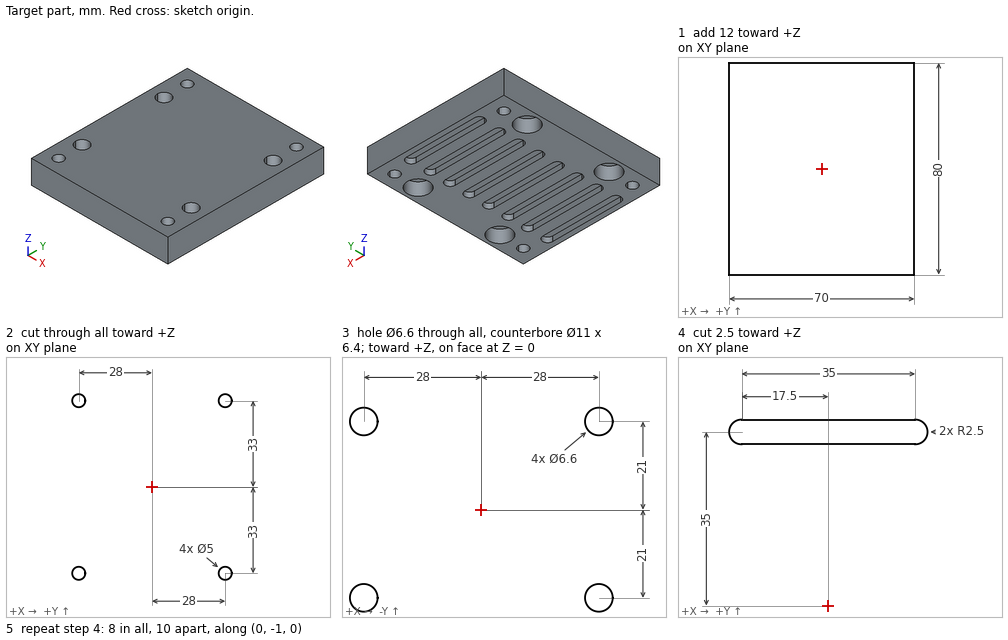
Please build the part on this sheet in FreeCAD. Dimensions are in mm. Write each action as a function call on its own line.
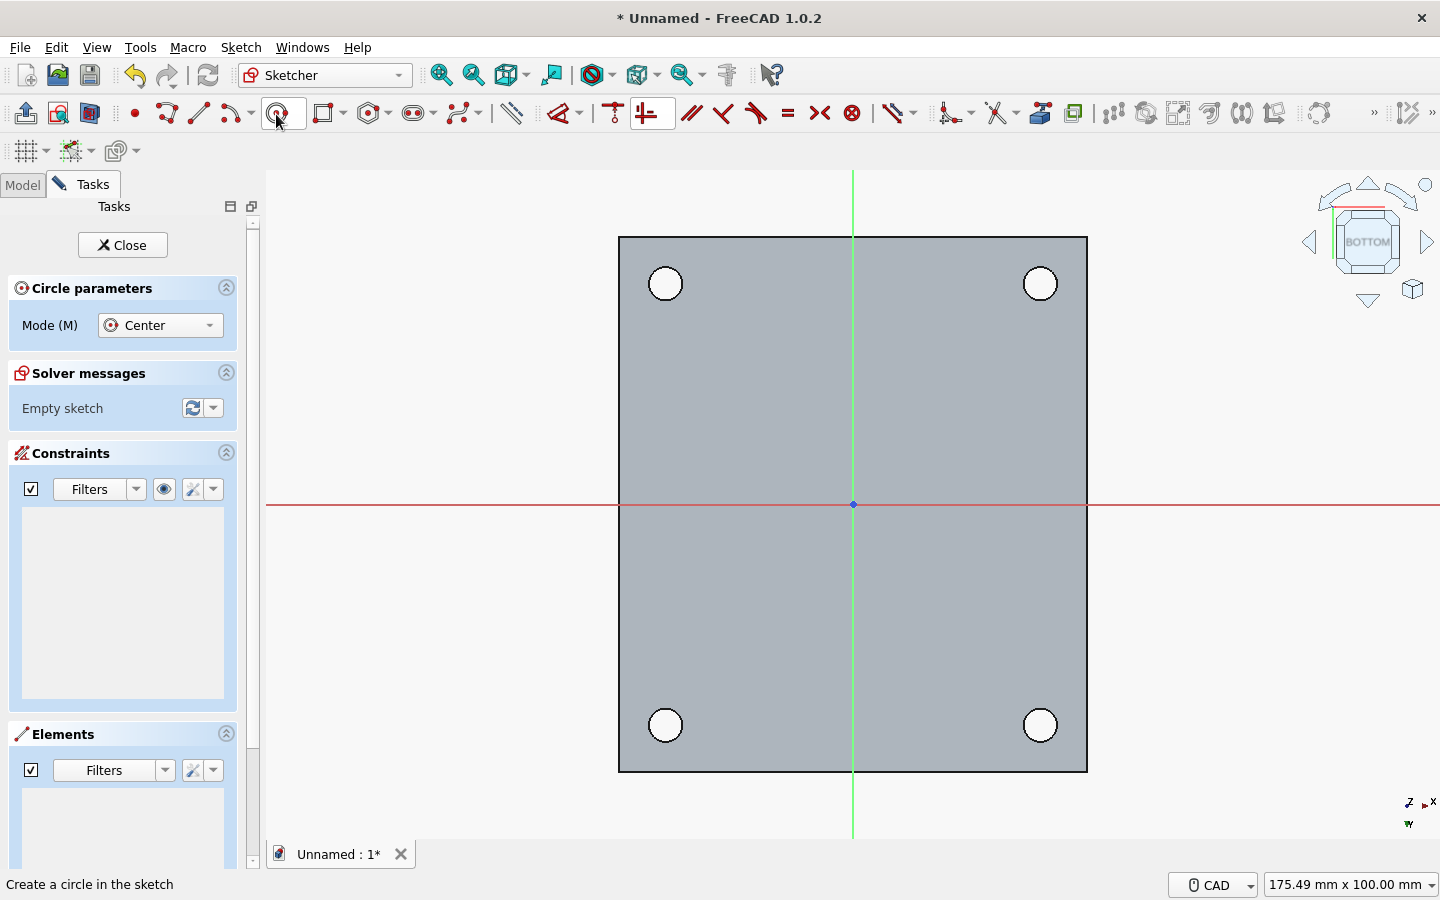
click(1040, 364)
move(1056, 348)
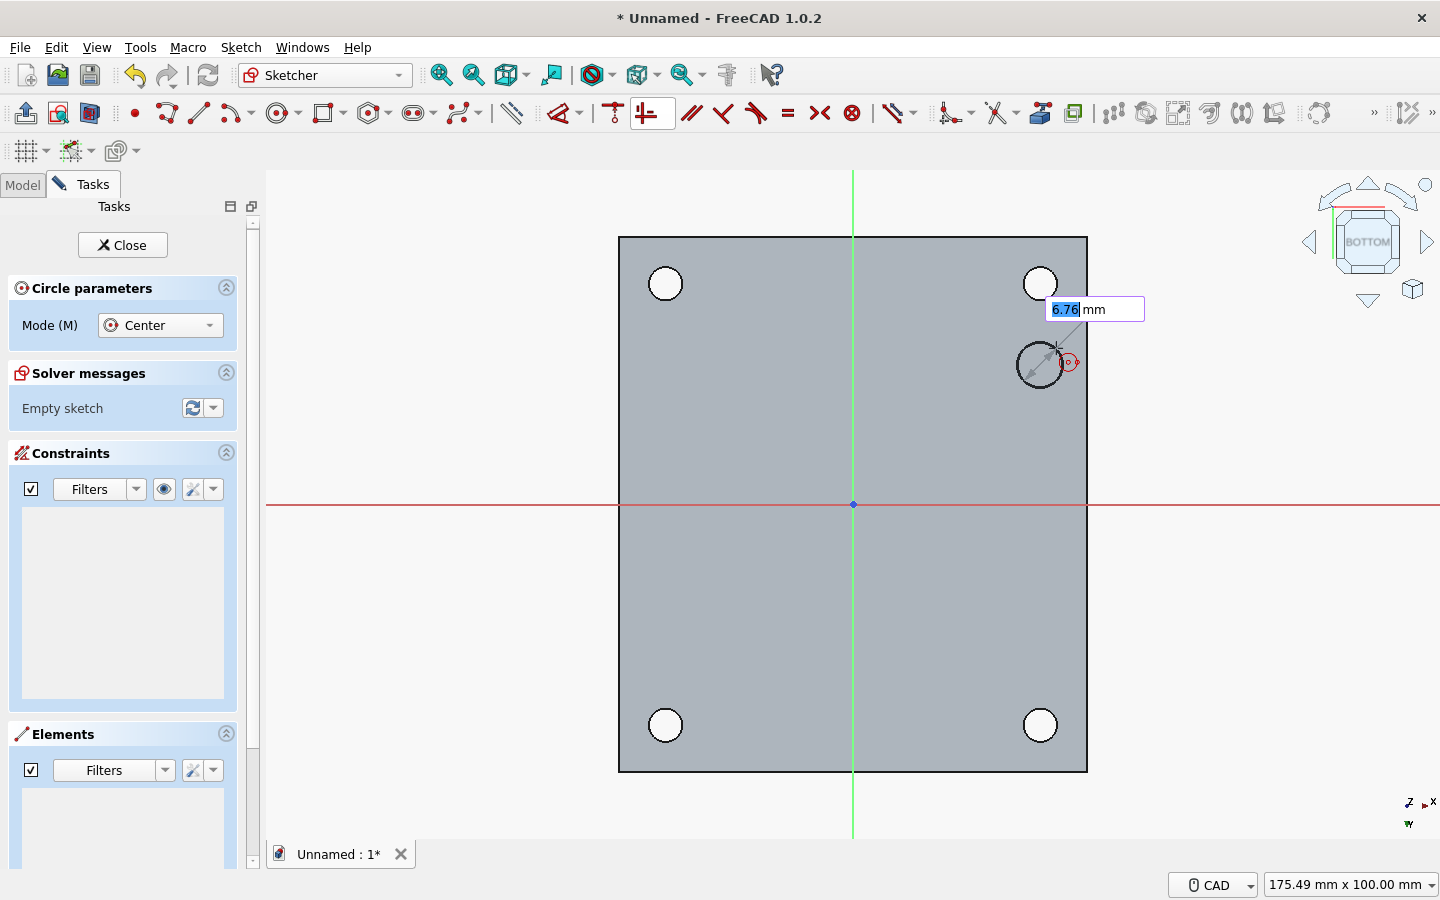
text(6.6)
key(Return)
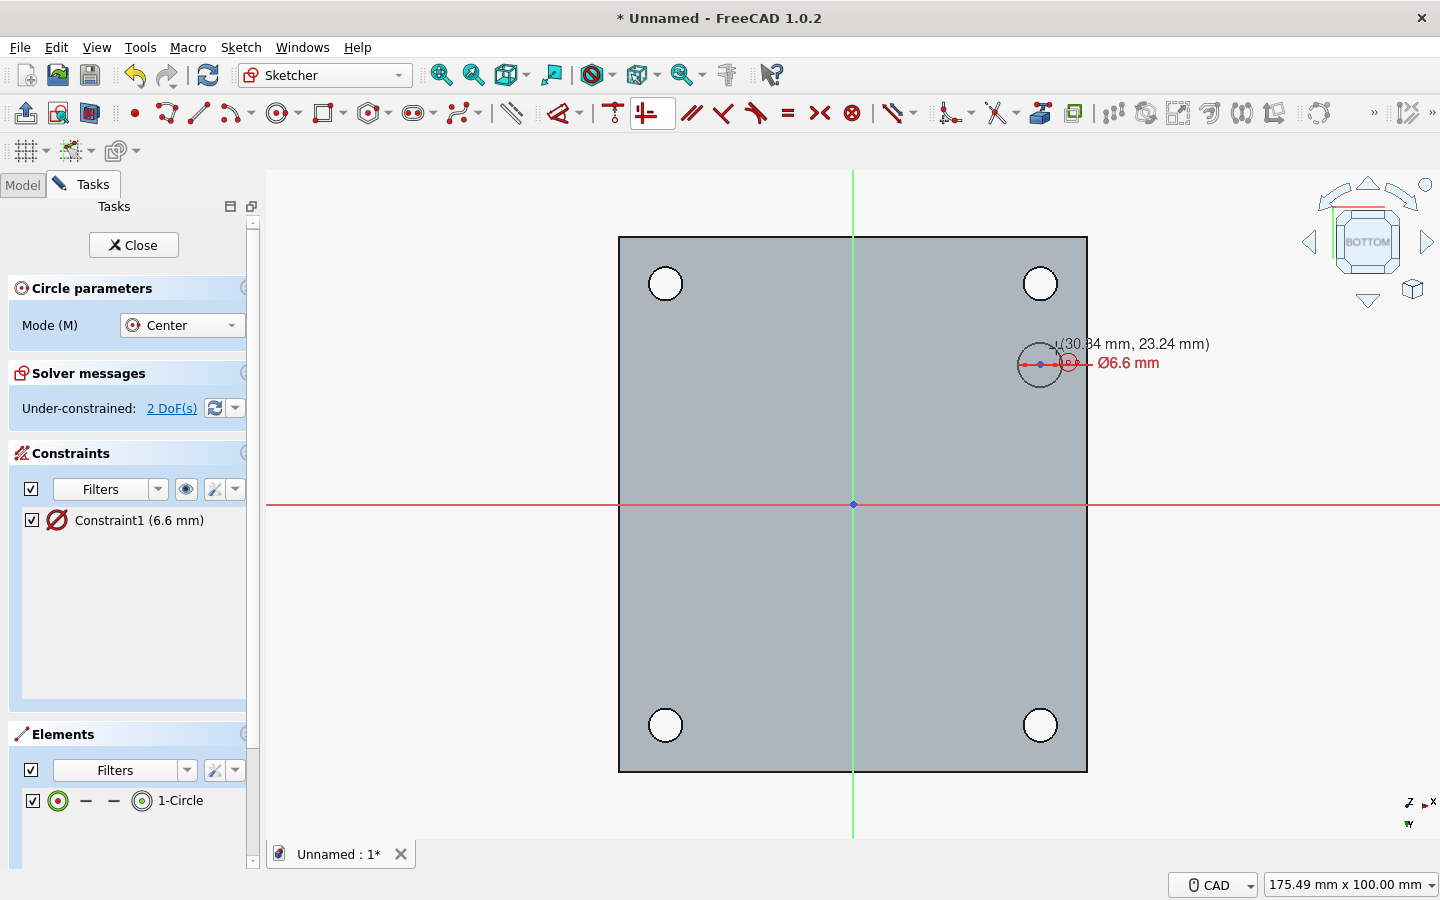
click(1040, 645)
move(1056, 629)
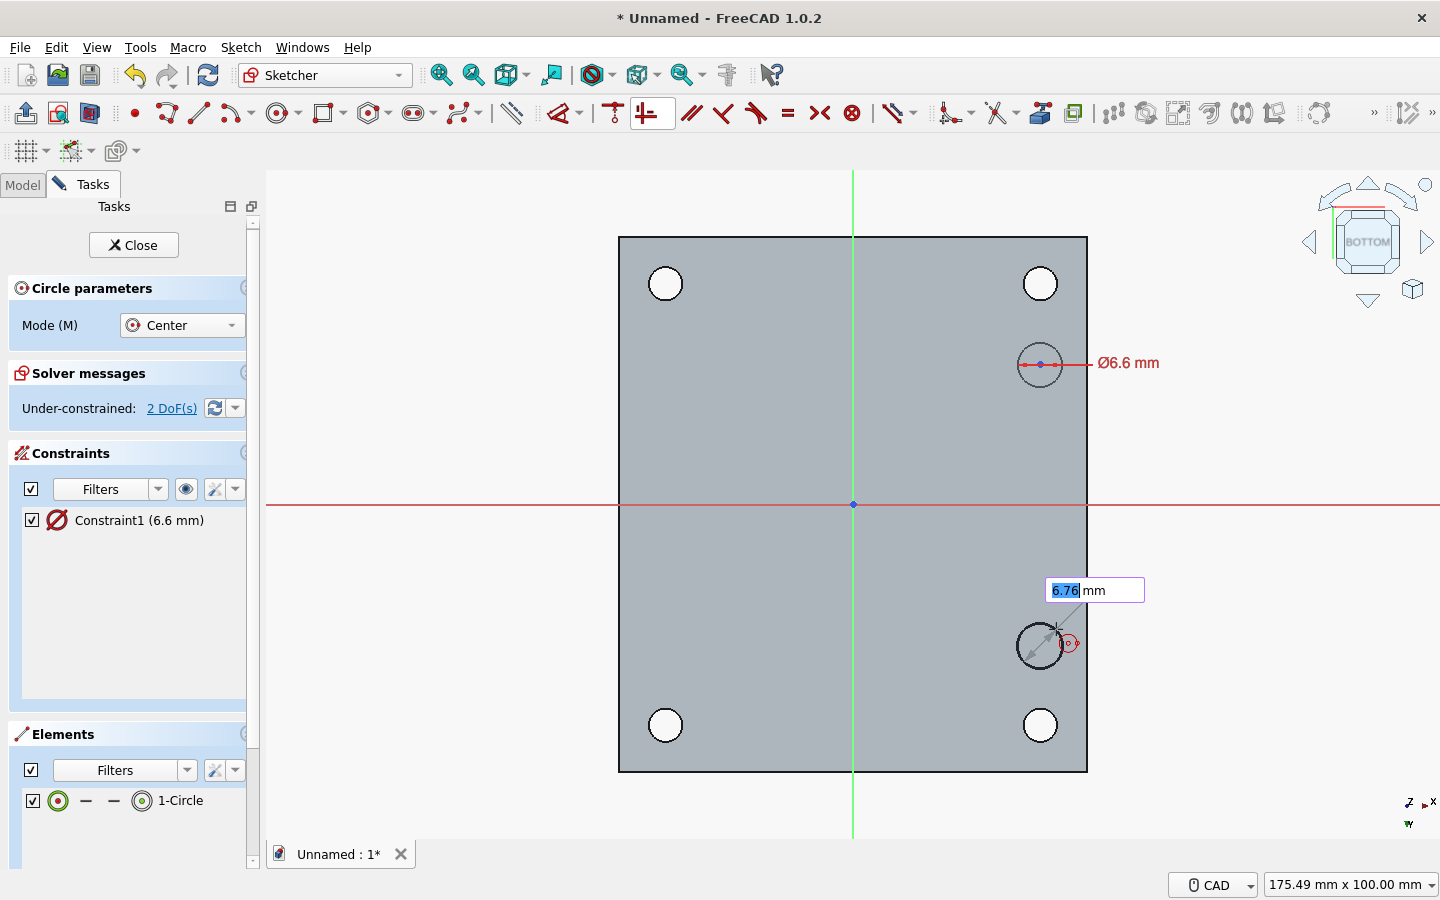
text(6.6)
key(Return)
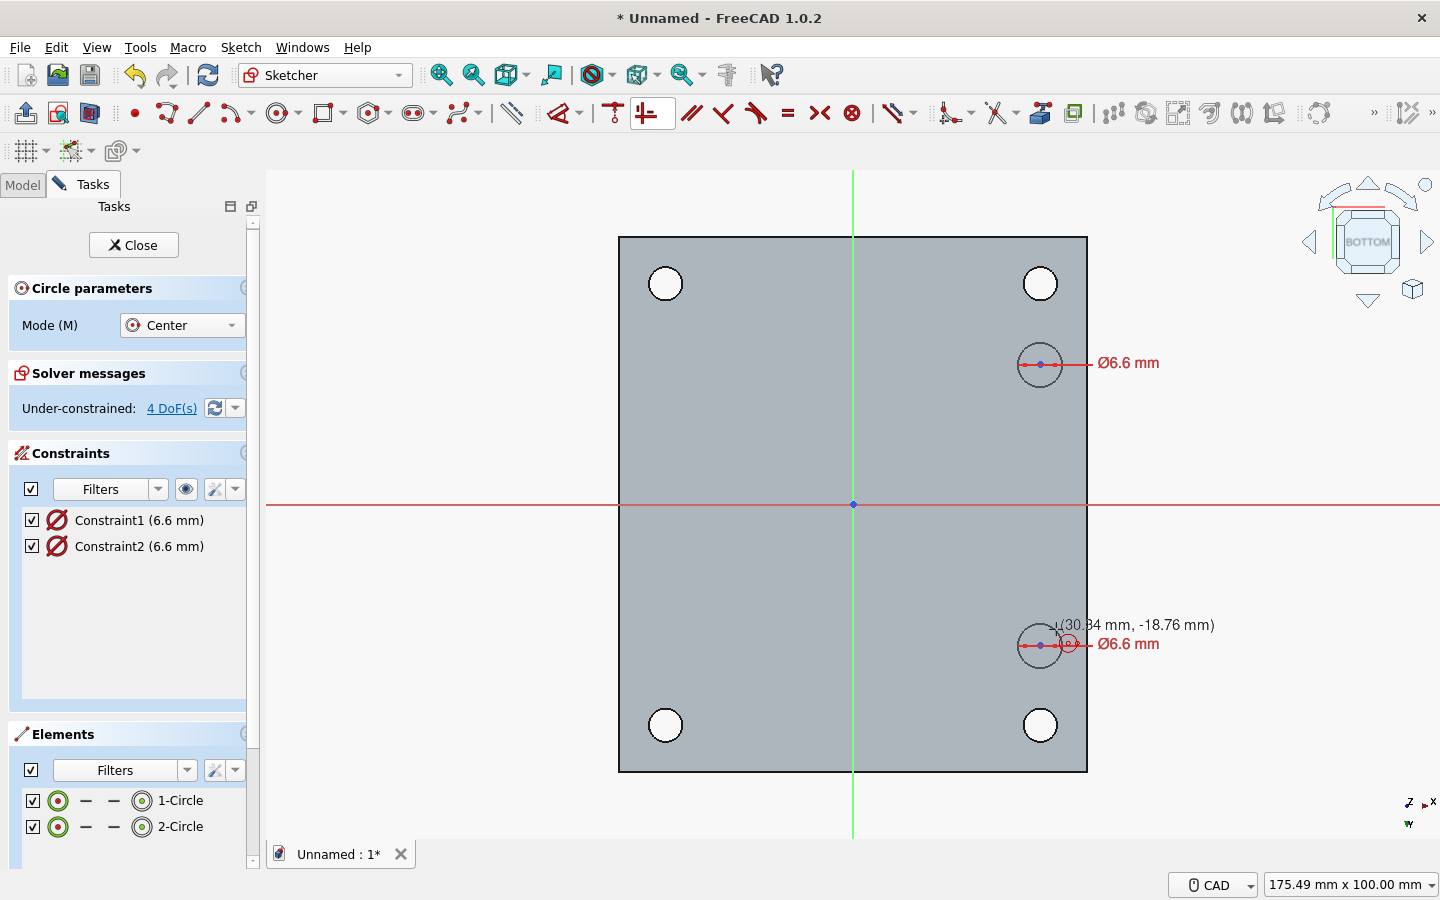
click(666, 364)
move(681, 348)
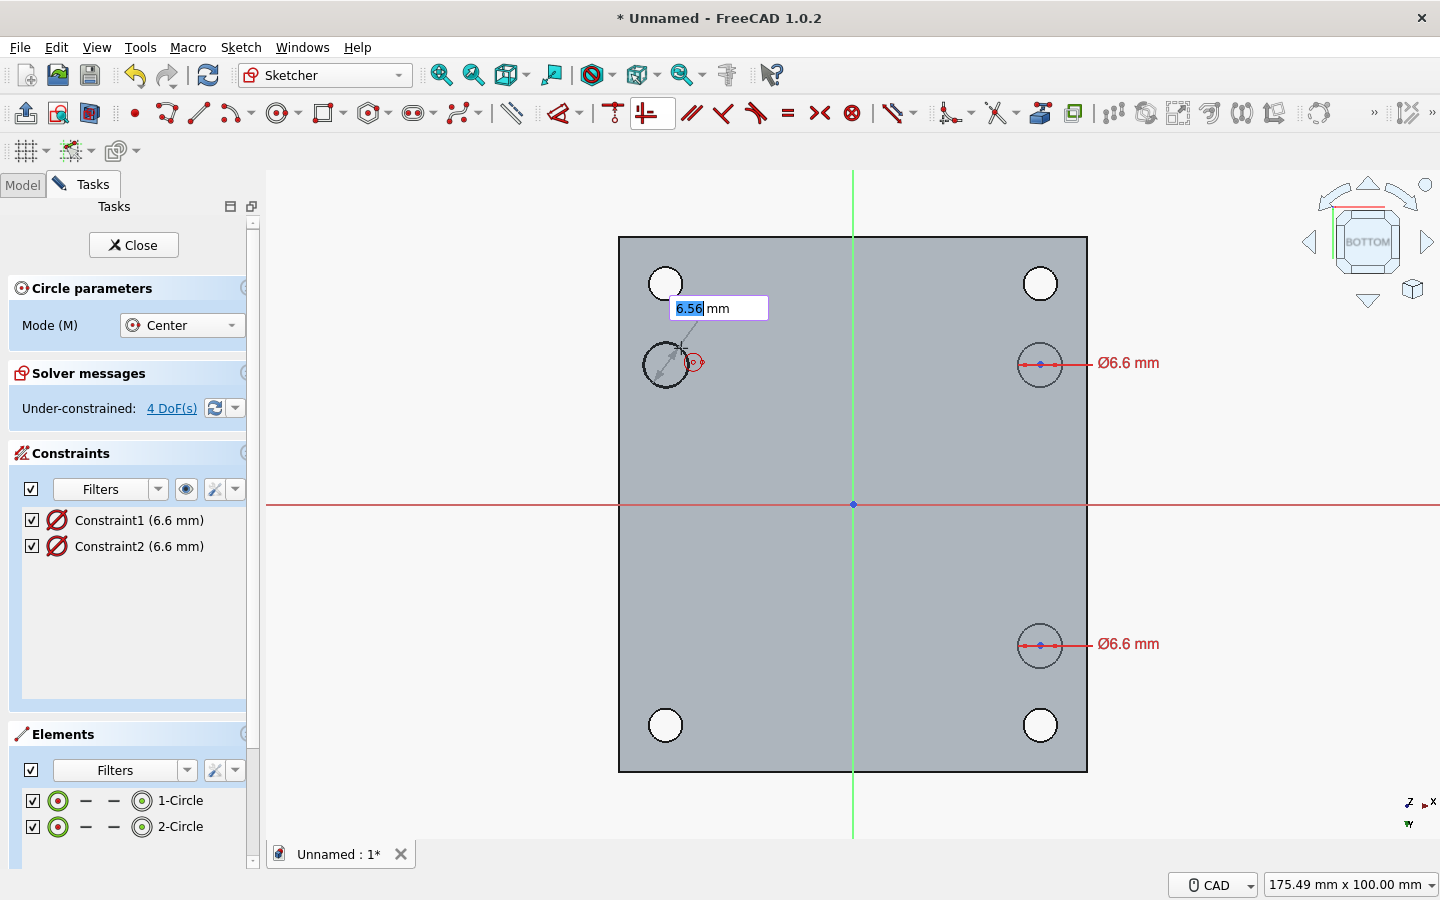
text(6.6)
key(Return)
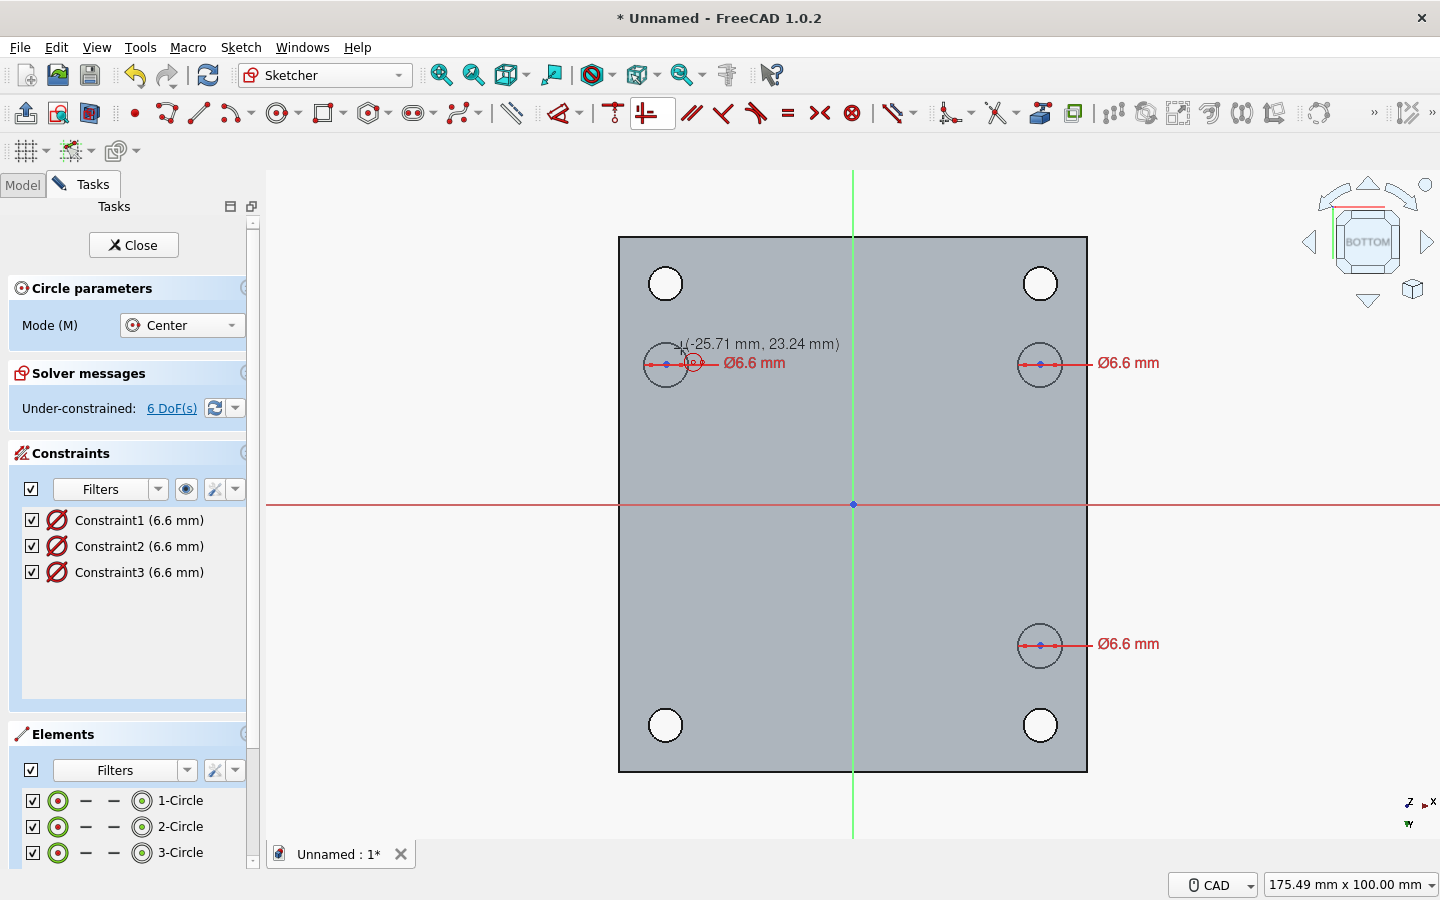
click(666, 645)
move(681, 629)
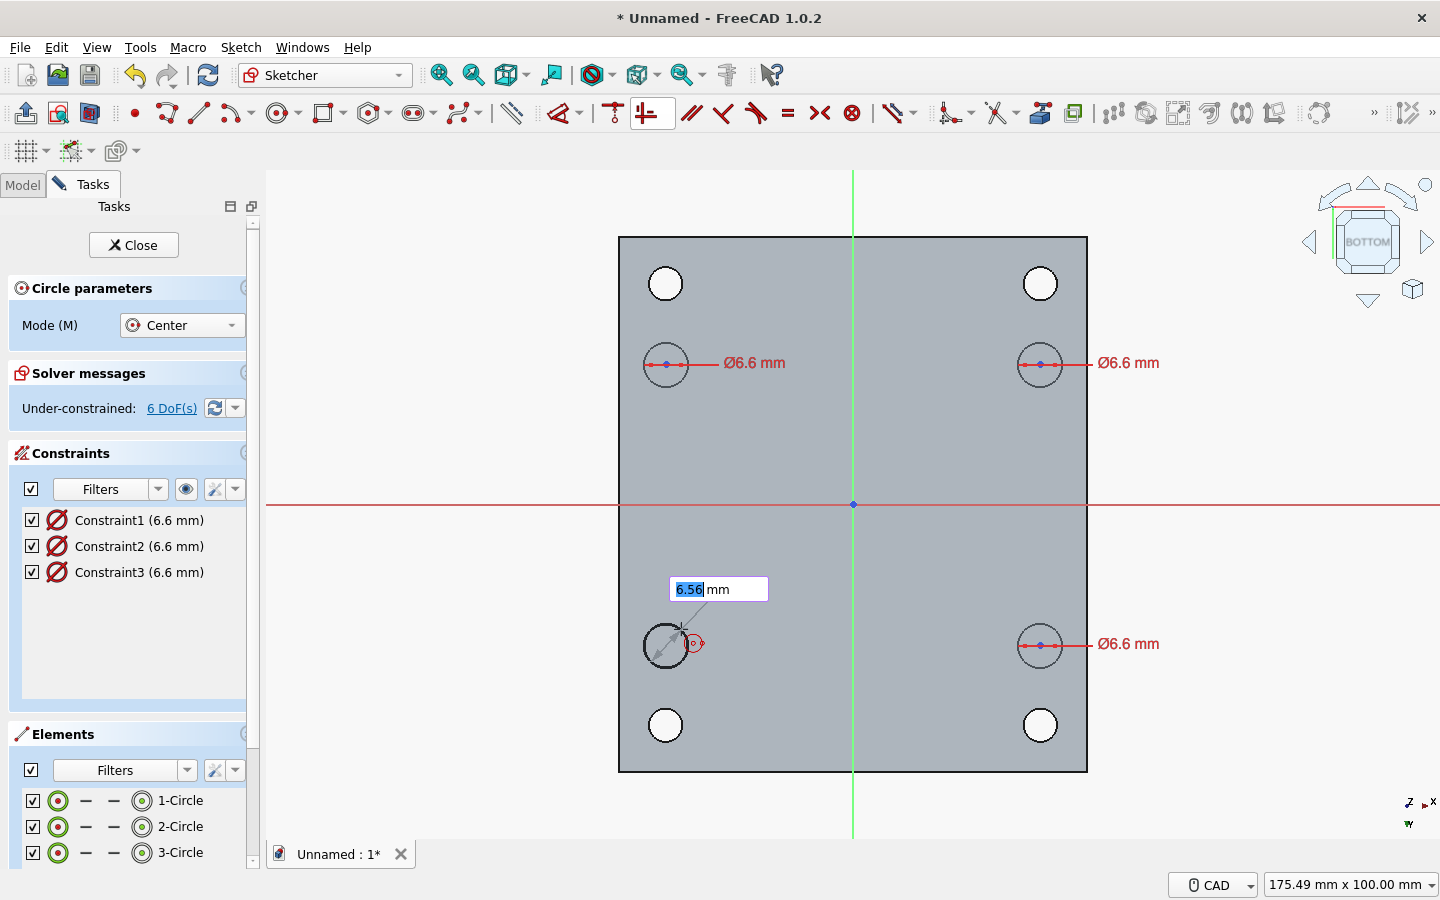
text(6.6)
key(Return)
key(Escape)